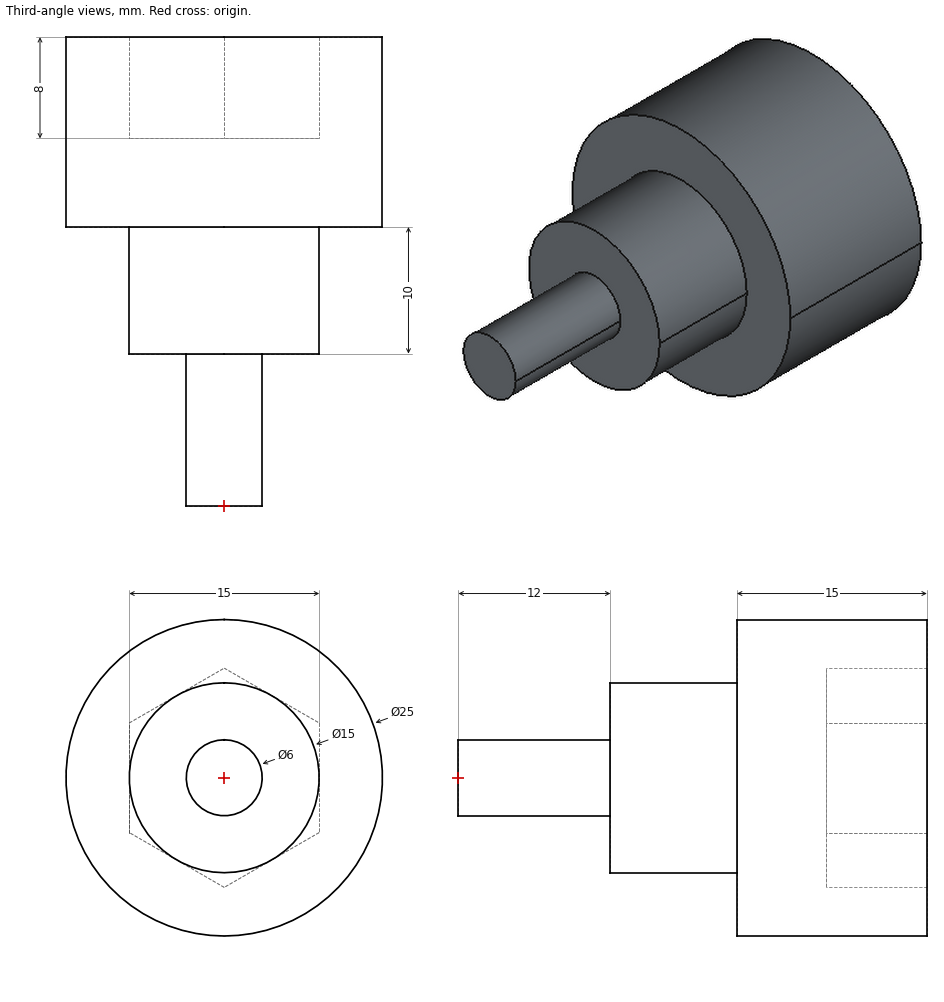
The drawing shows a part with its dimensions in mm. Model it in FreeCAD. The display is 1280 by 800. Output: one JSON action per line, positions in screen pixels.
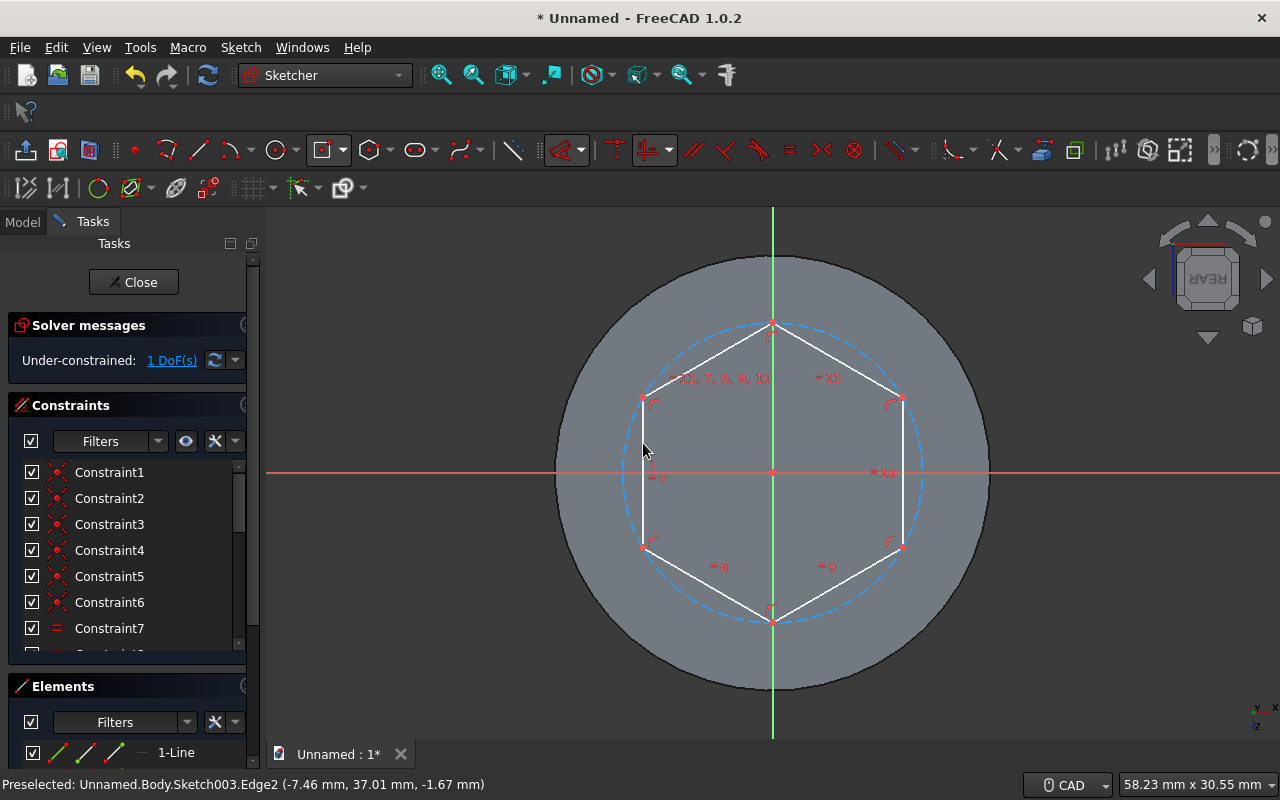
{"action": "left_click", "coordinate": [643, 398]}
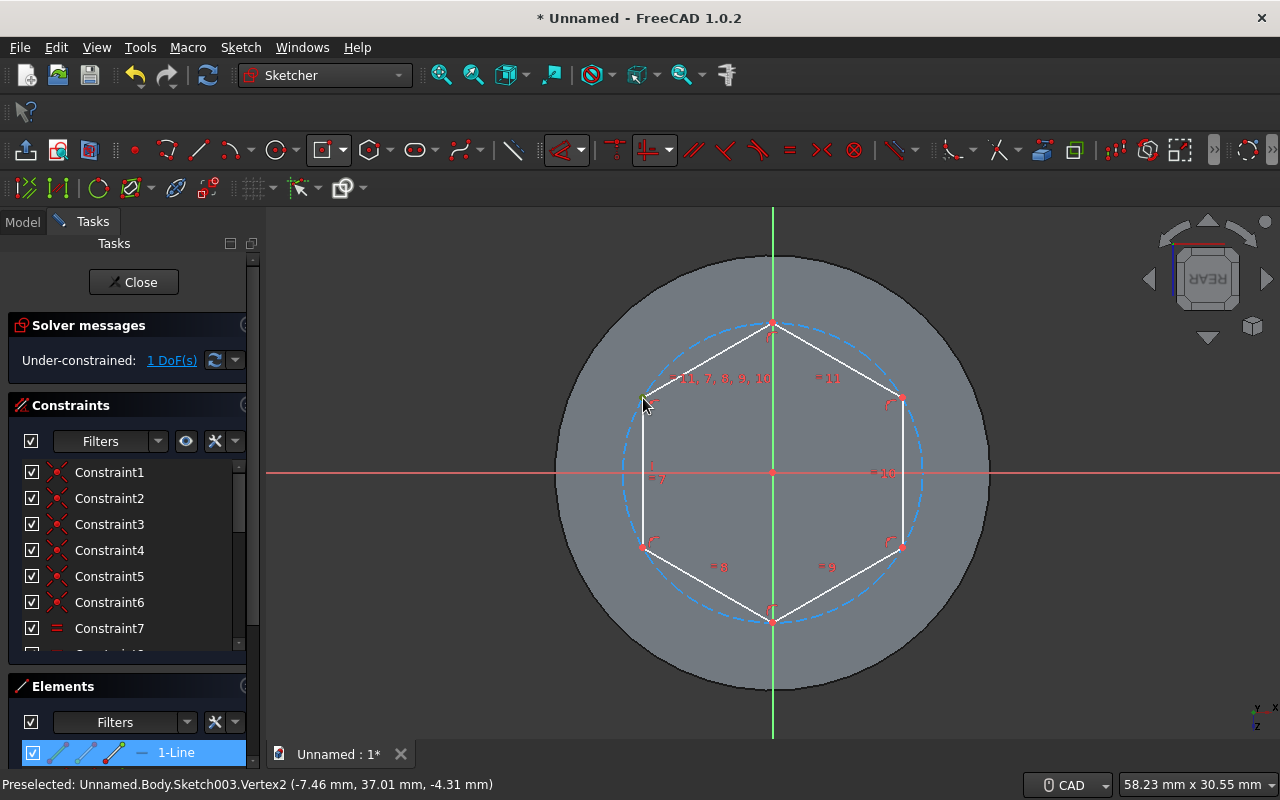
{"action": "left_click", "coordinate": [903, 548]}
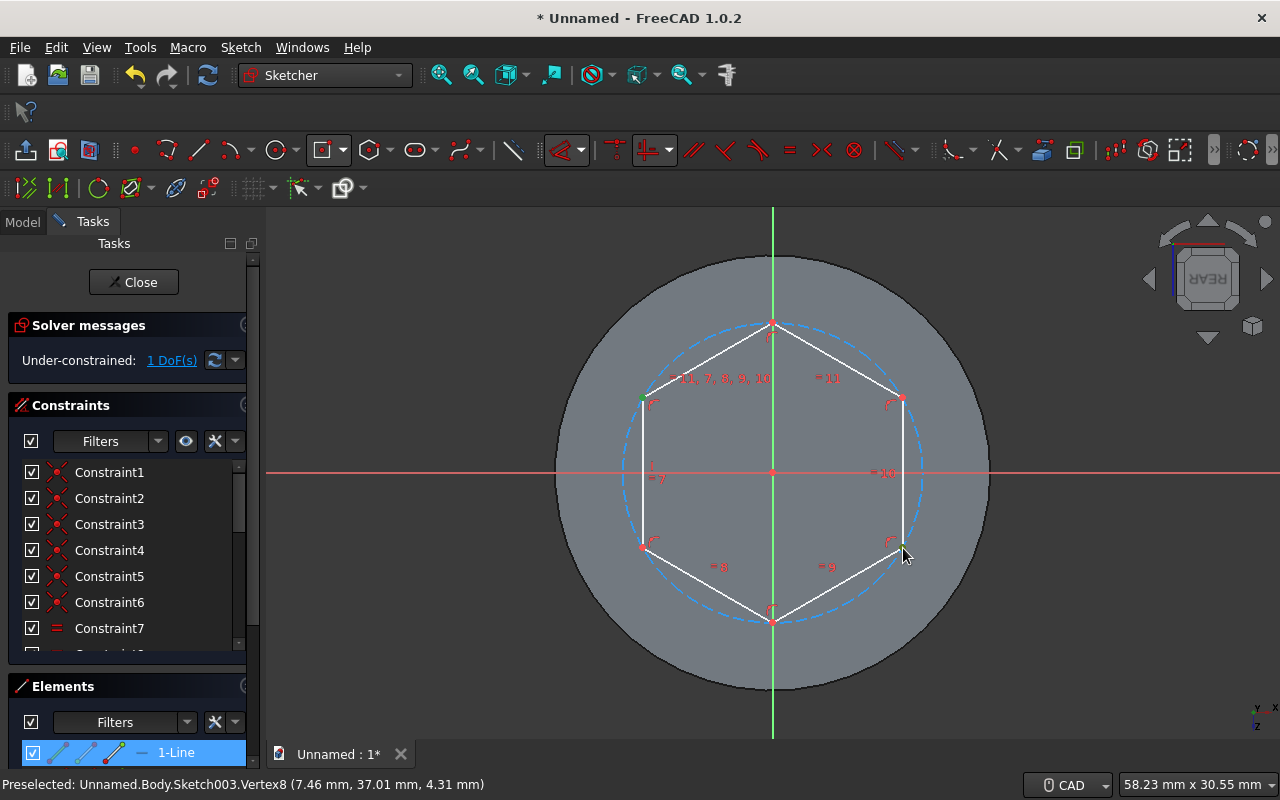
{"action": "key", "text": "l"}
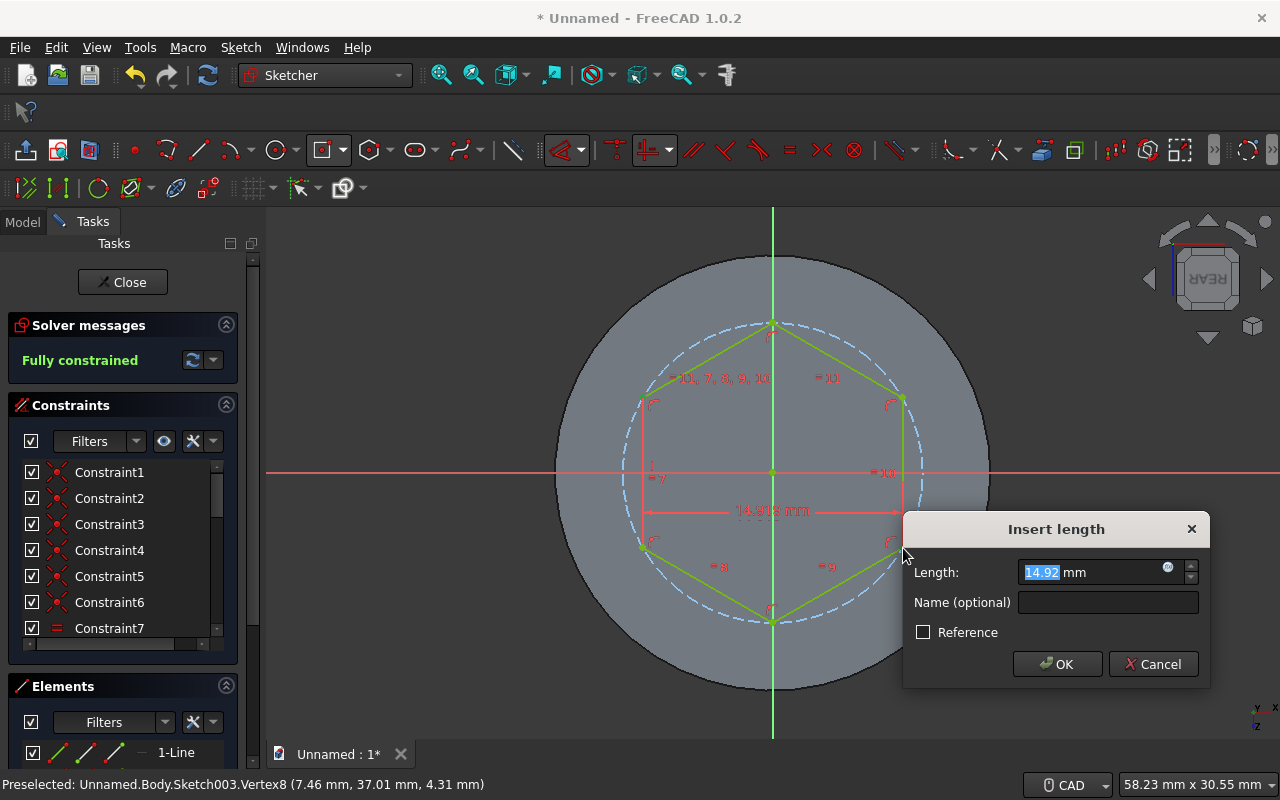
{"action": "type", "text": "15"}
{"action": "key", "text": "Return"}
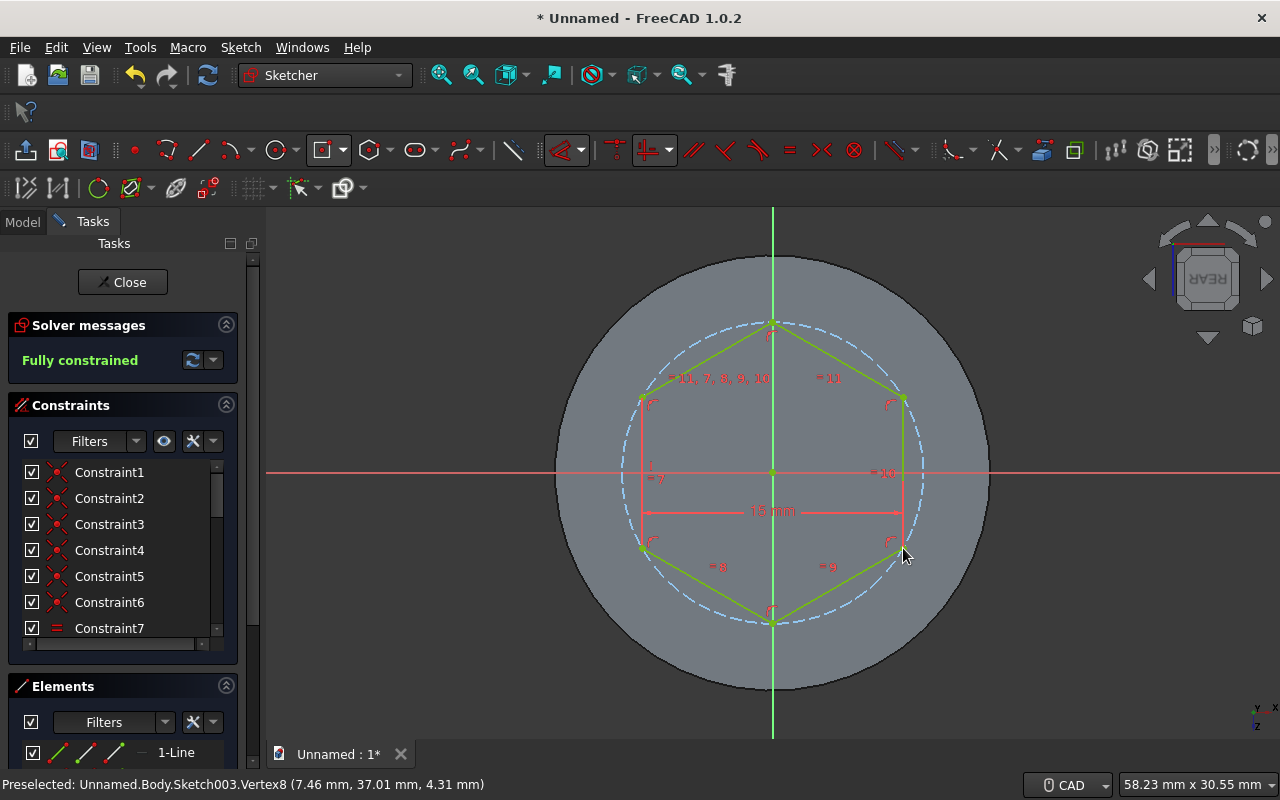
{"action": "left_click", "coordinate": [123, 282]}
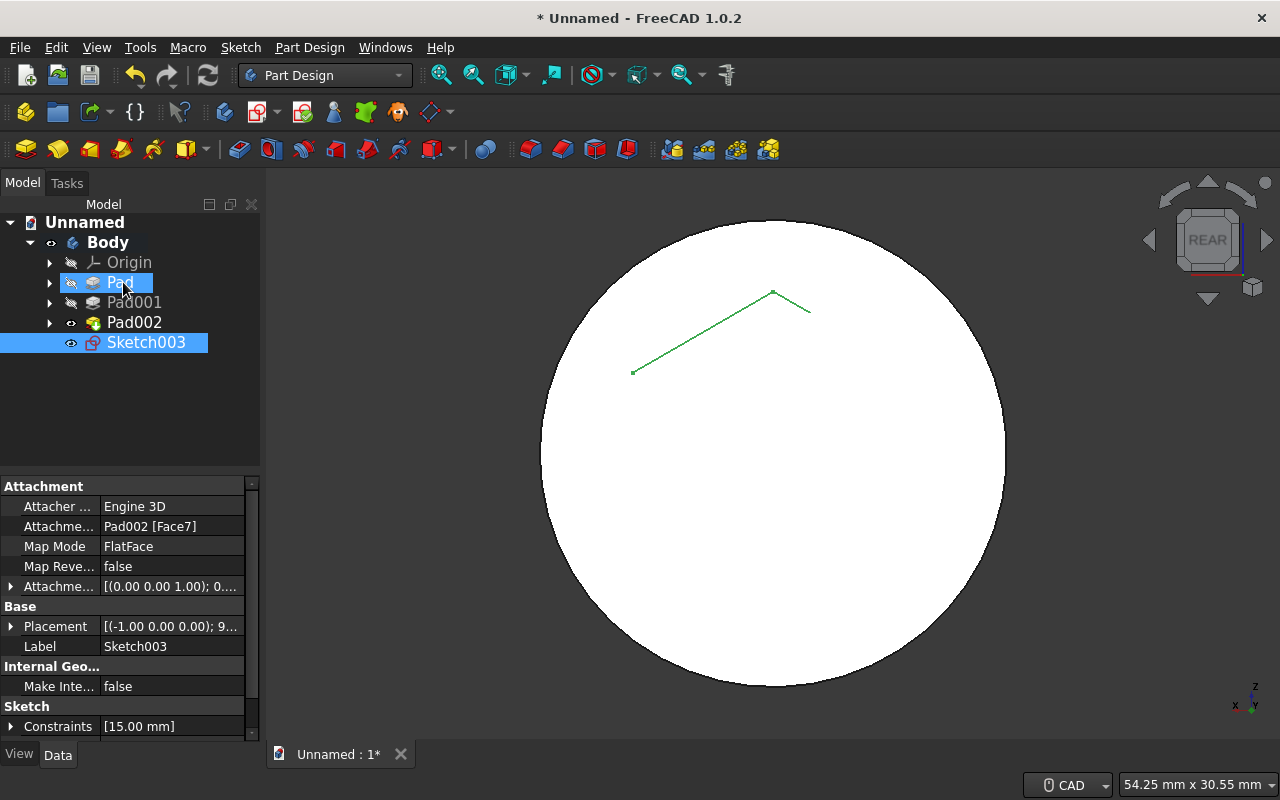
{"action": "left_click", "coordinate": [240, 150]}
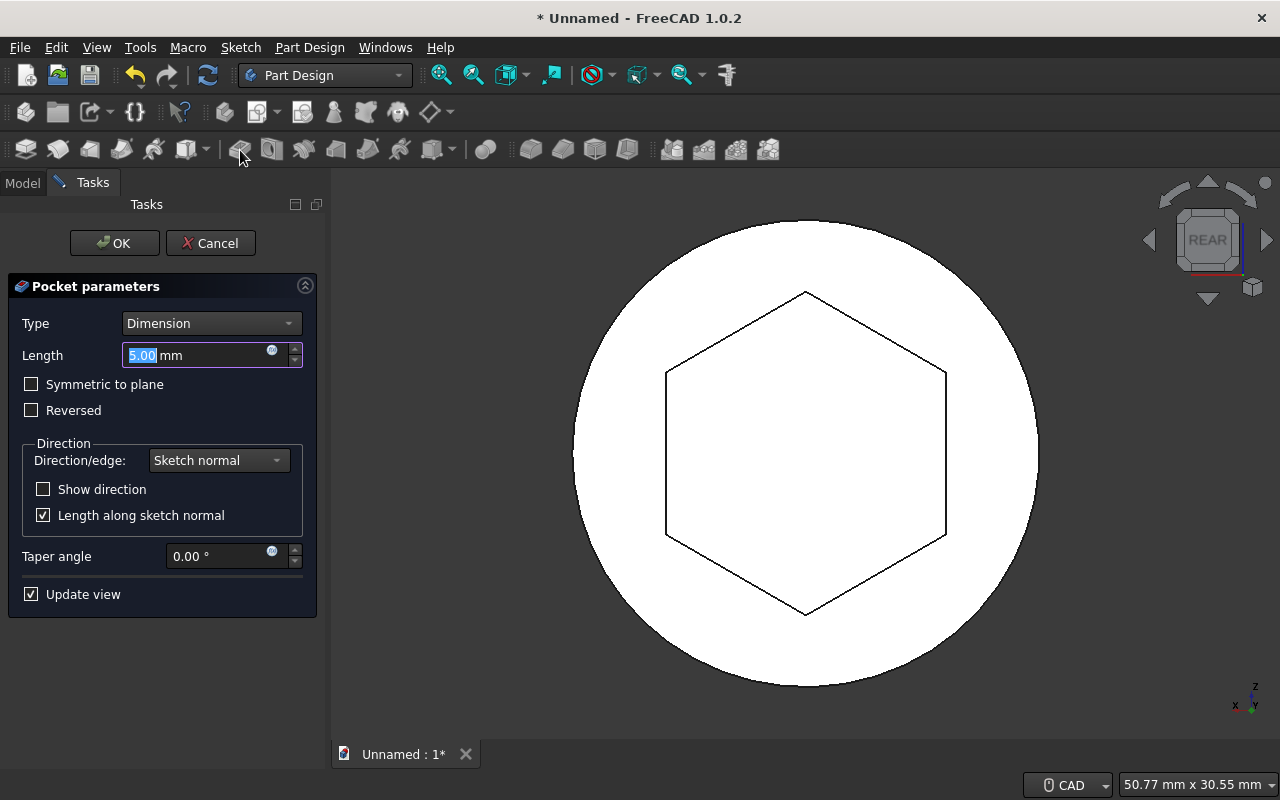
{"action": "type", "text": "8"}
{"action": "key", "text": "Tab"}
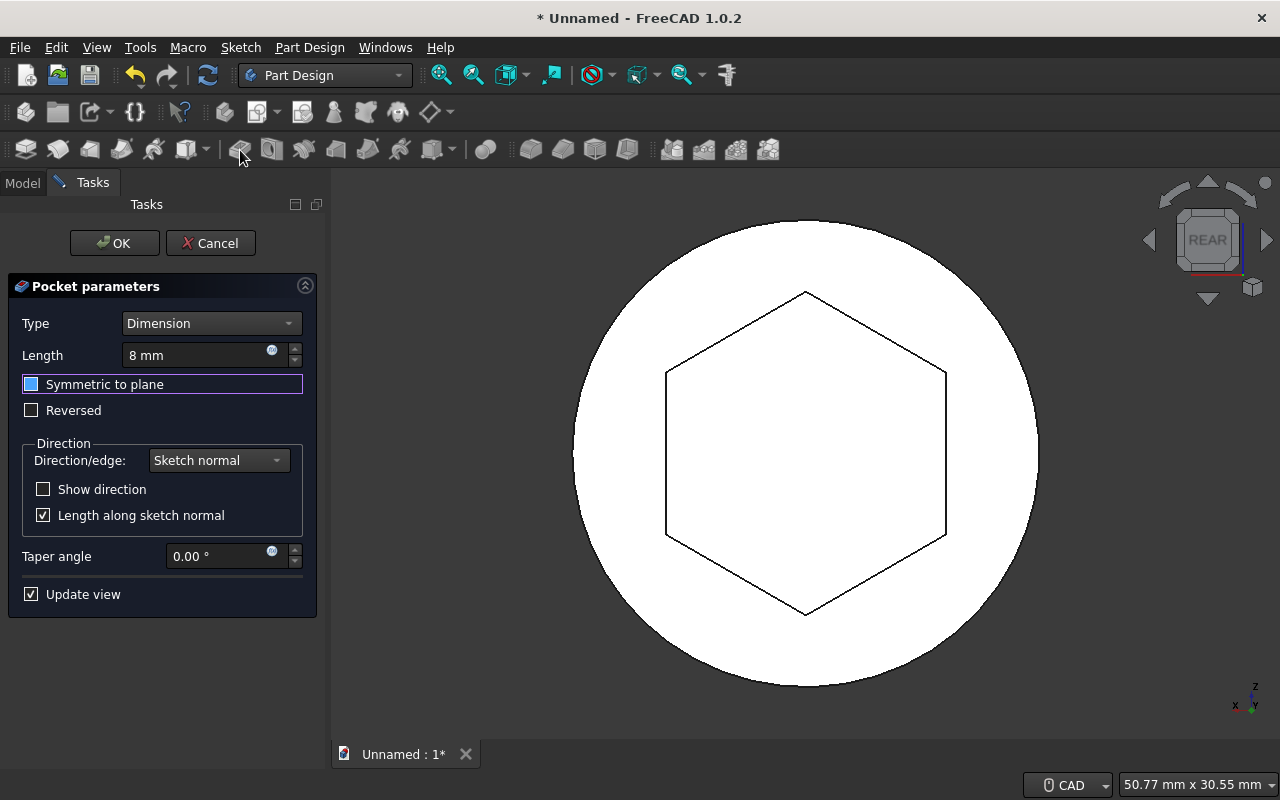
{"action": "left_click", "coordinate": [115, 243]}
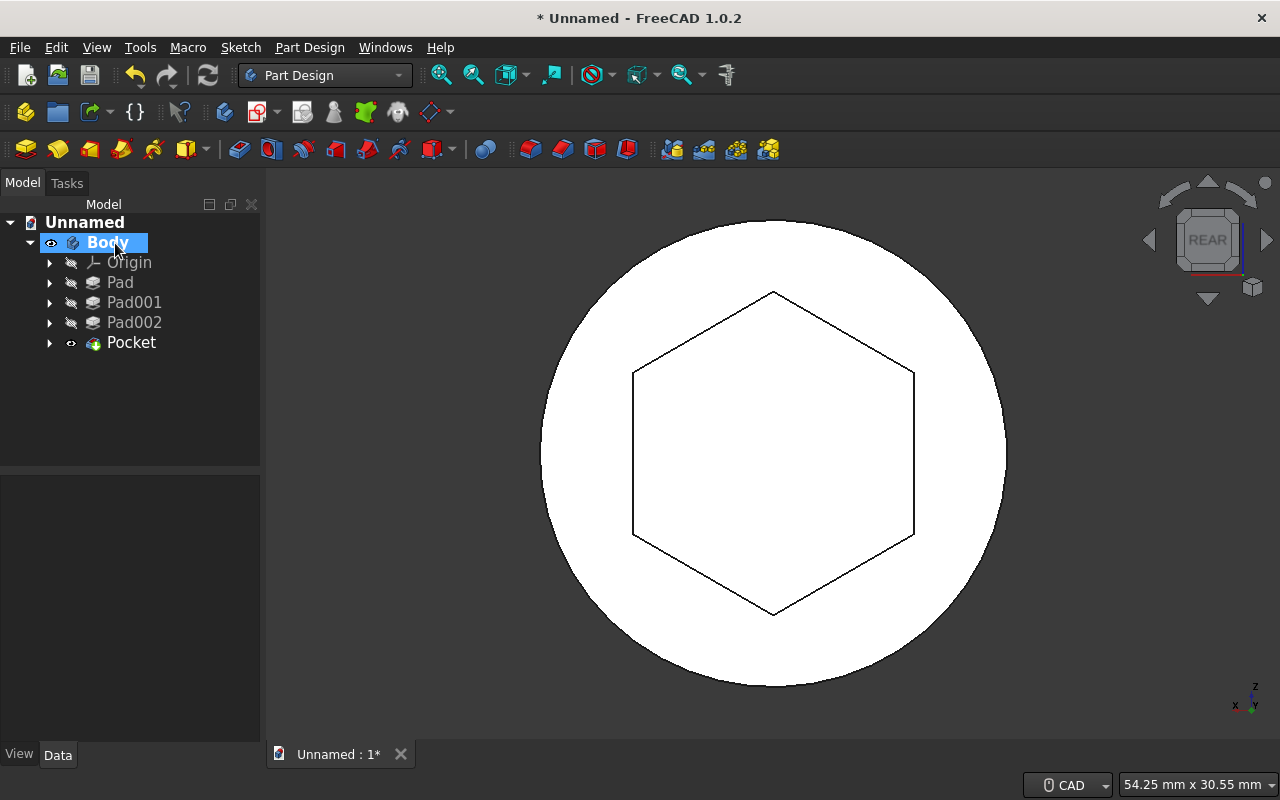
{"action": "key", "text": "0"}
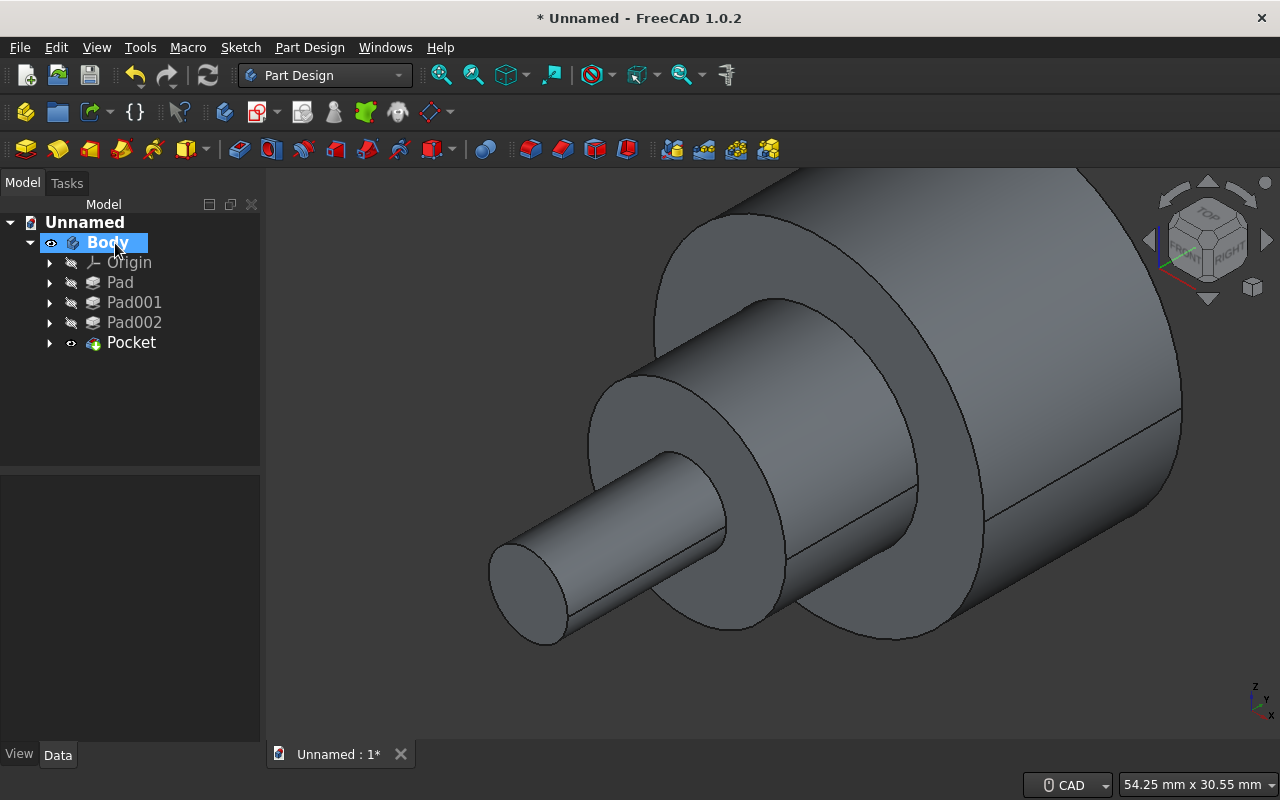
{"action": "left_click", "coordinate": [442, 76]}